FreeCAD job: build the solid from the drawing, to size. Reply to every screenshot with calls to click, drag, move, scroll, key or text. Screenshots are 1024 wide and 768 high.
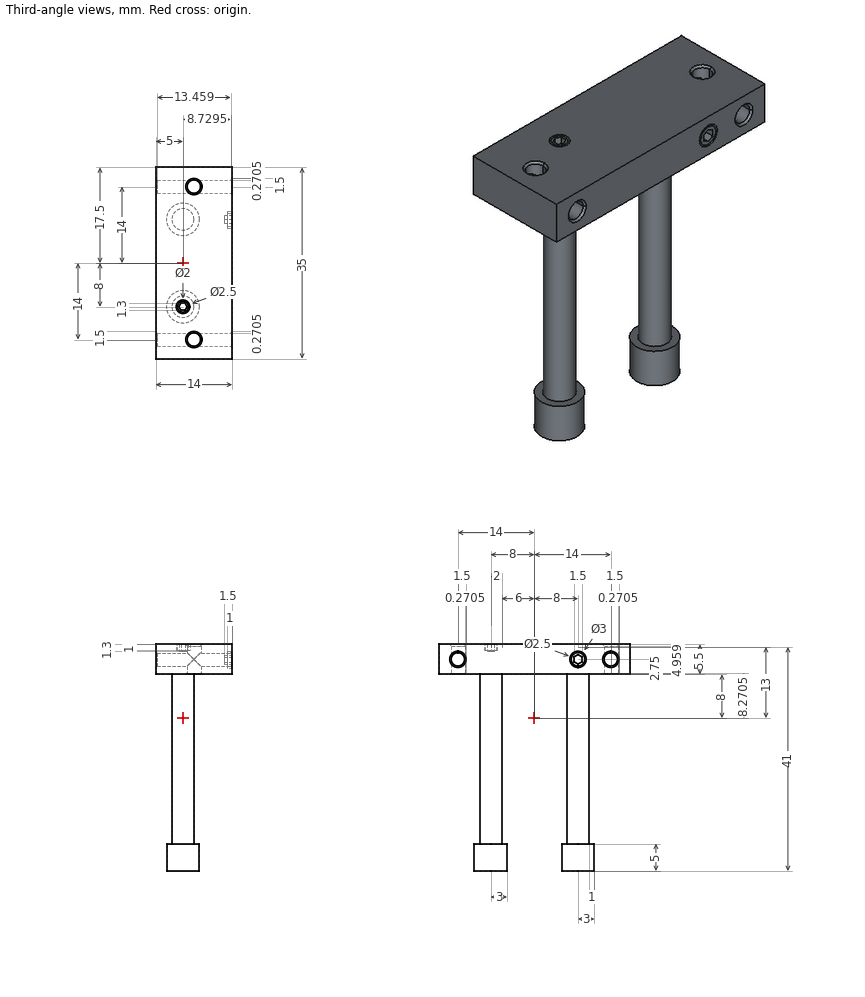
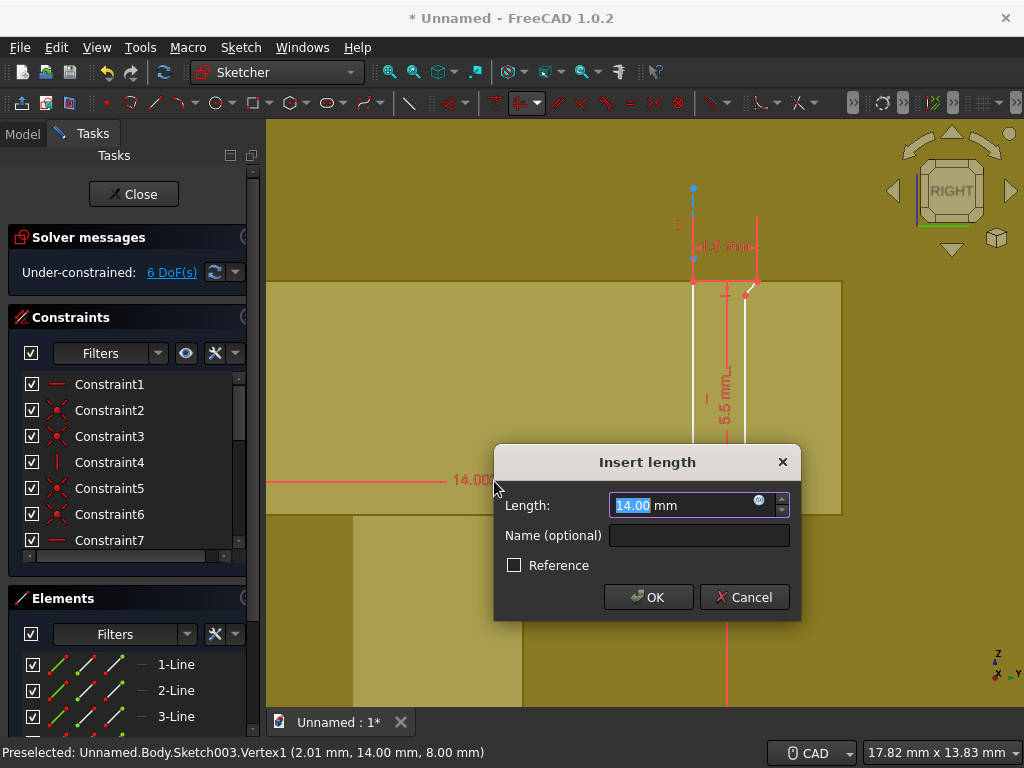
text(14)
key(Return)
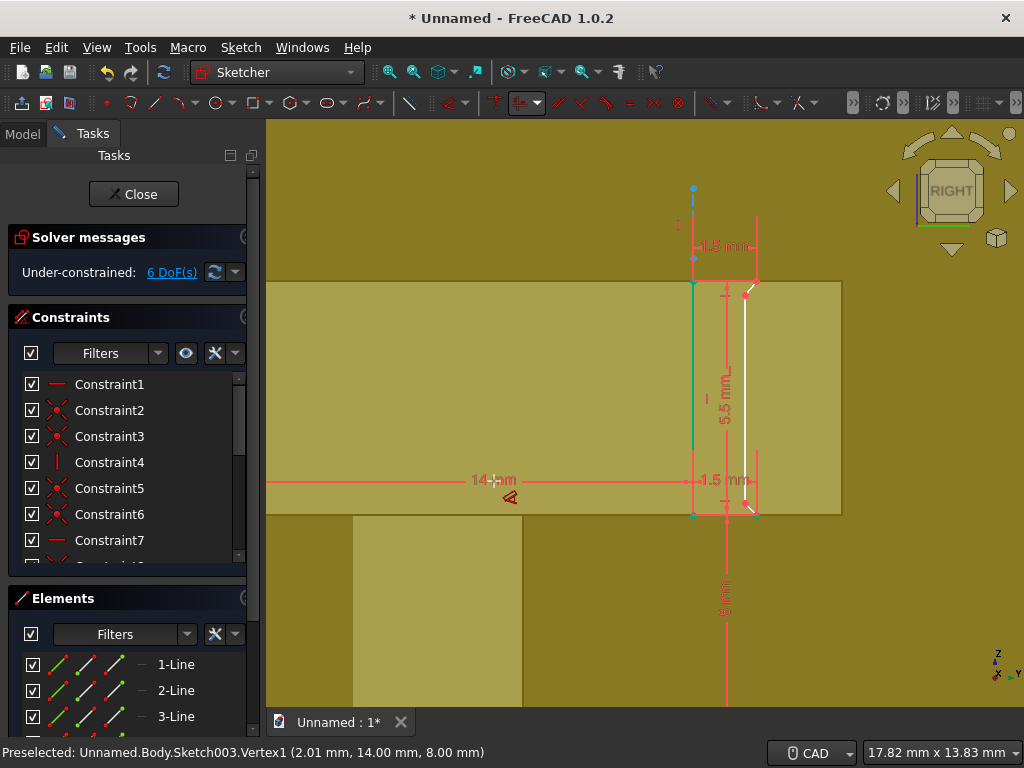
click(693, 259)
click(493, 225)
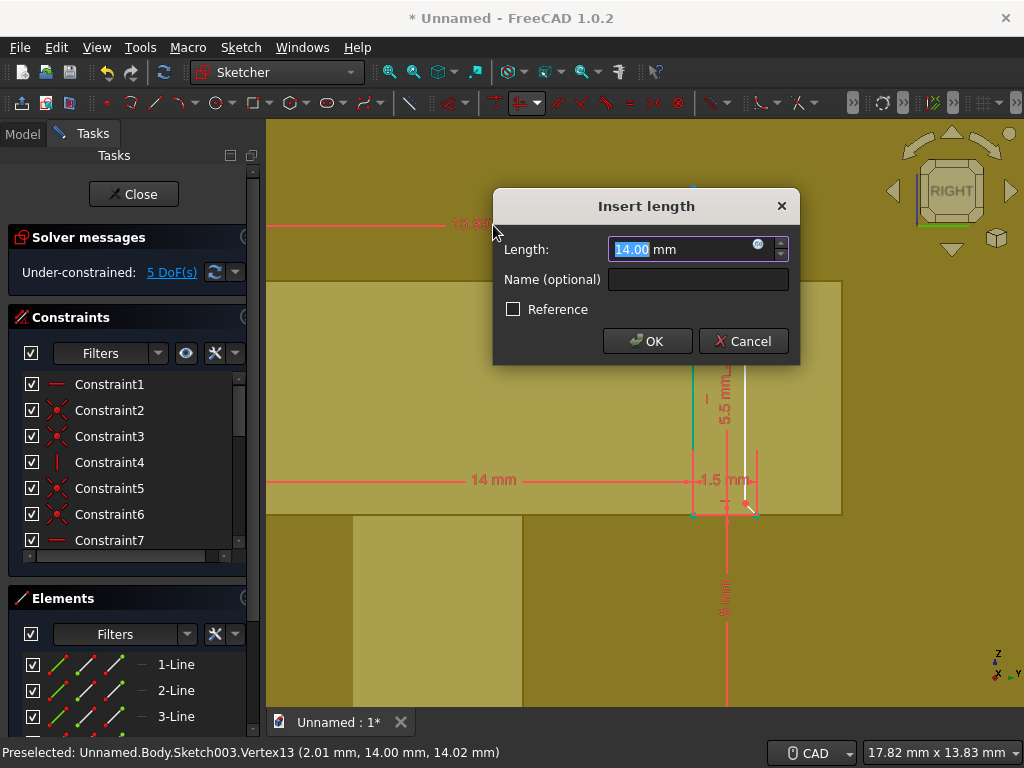
text(14)
key(Return)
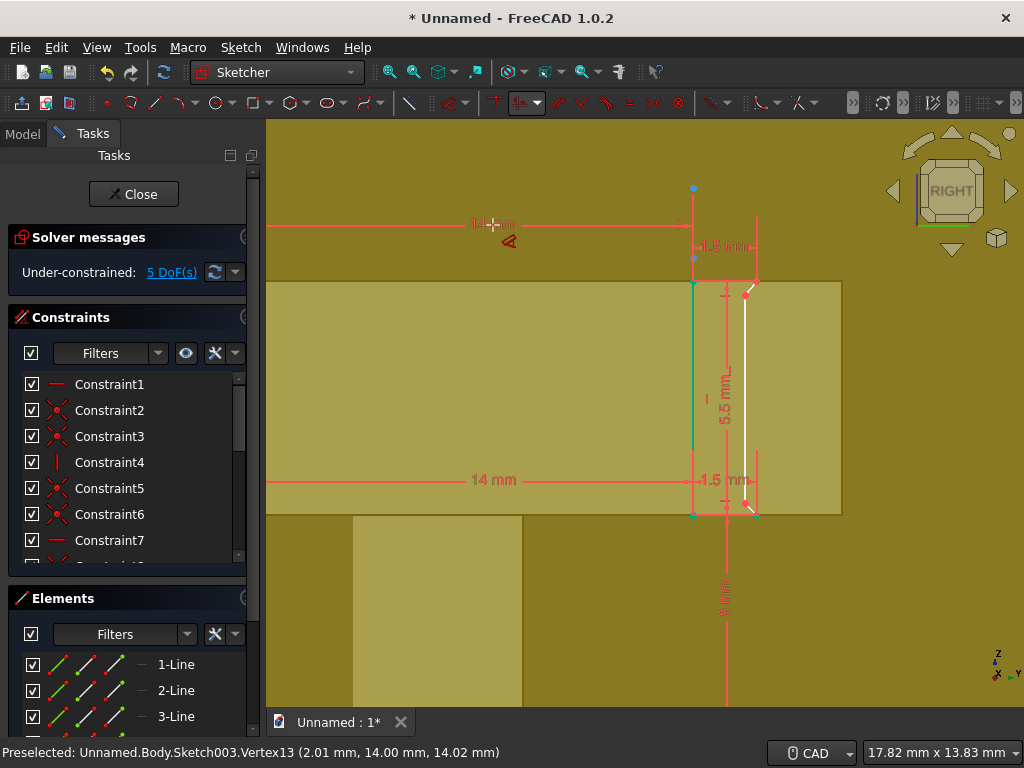
click(745, 441)
click(779, 352)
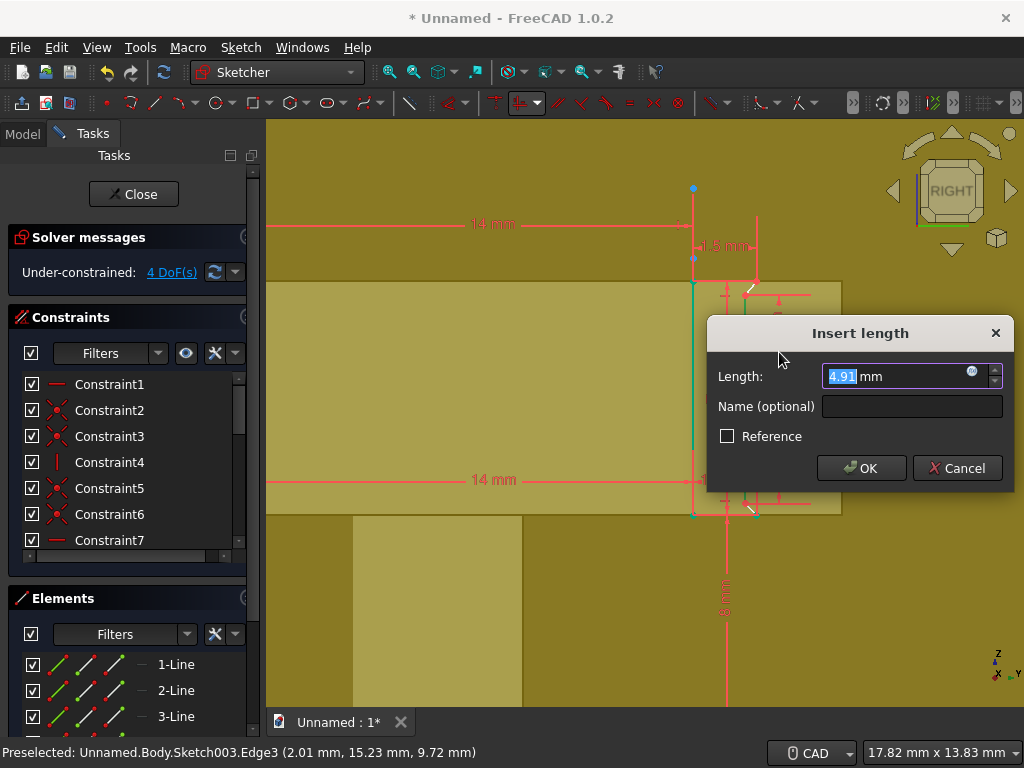
text(4.959)
key(Return)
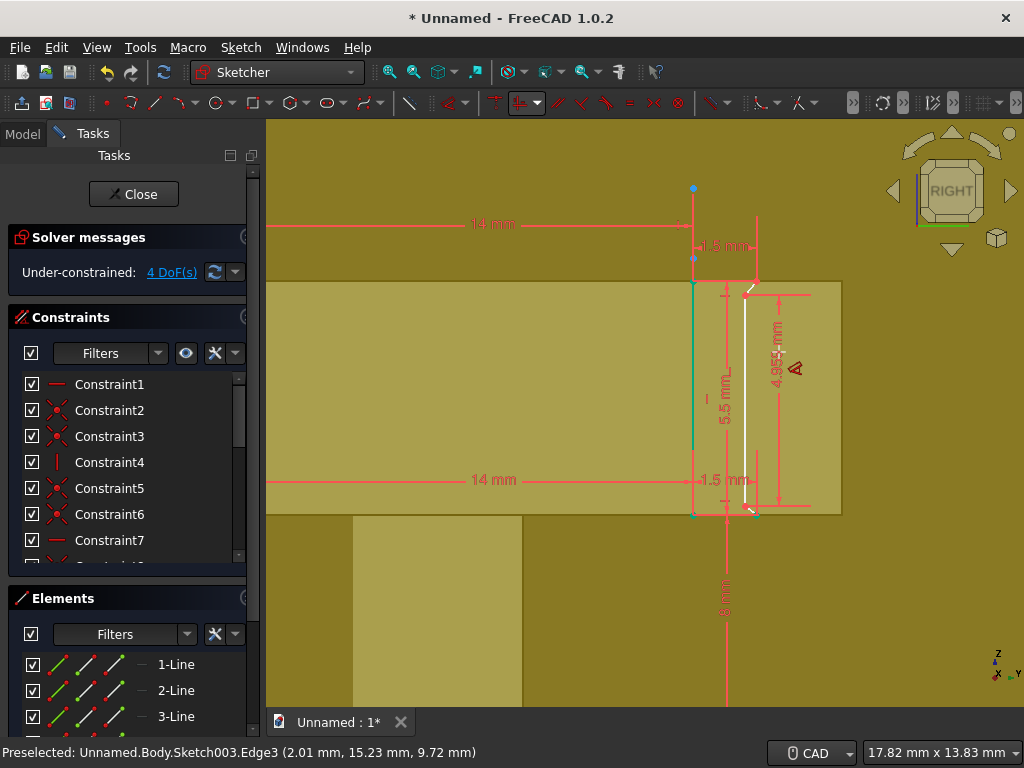
click(745, 506)
click(779, 553)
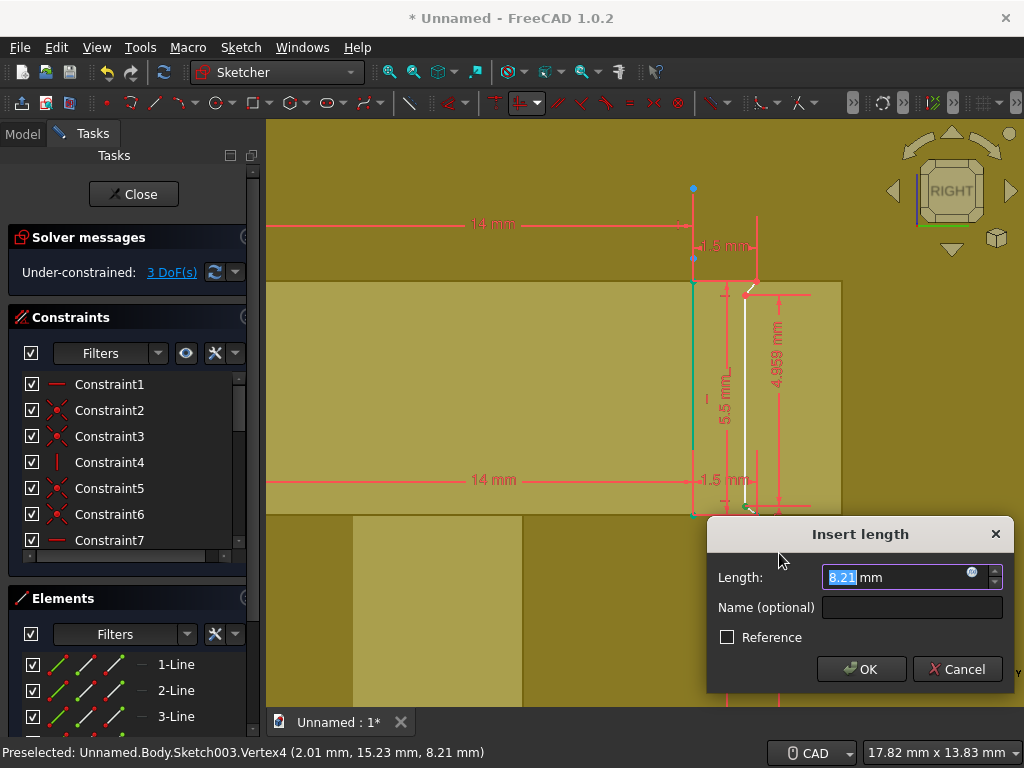
text(8.2705)
key(Return)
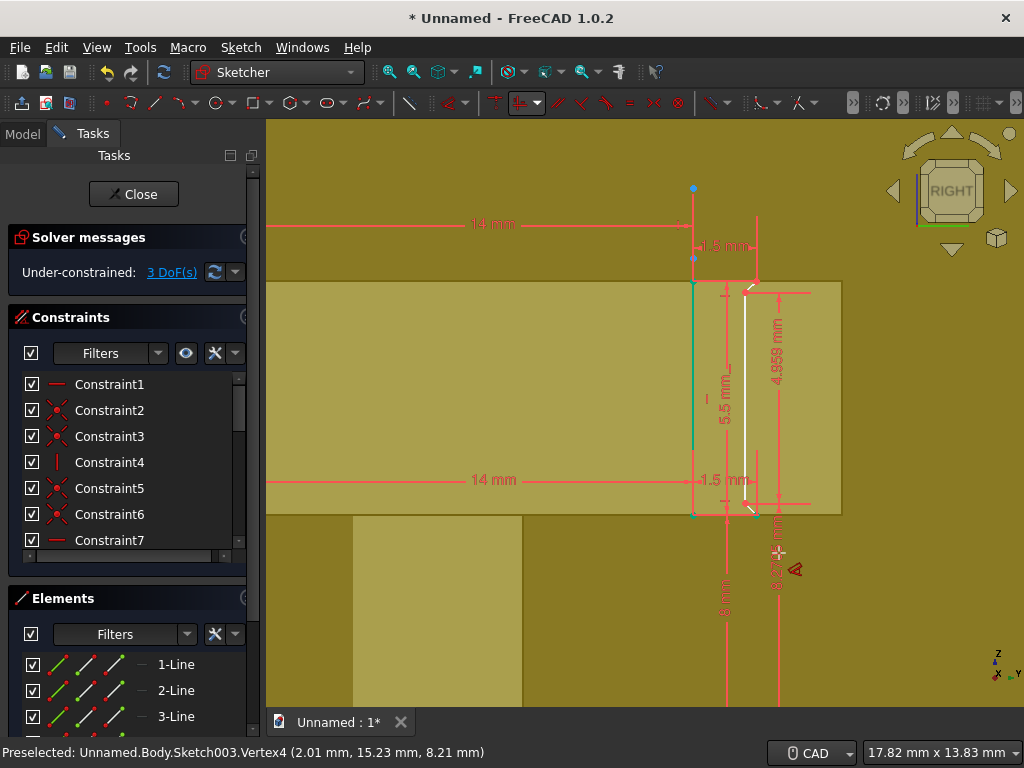
scroll(750, 508, up, 7)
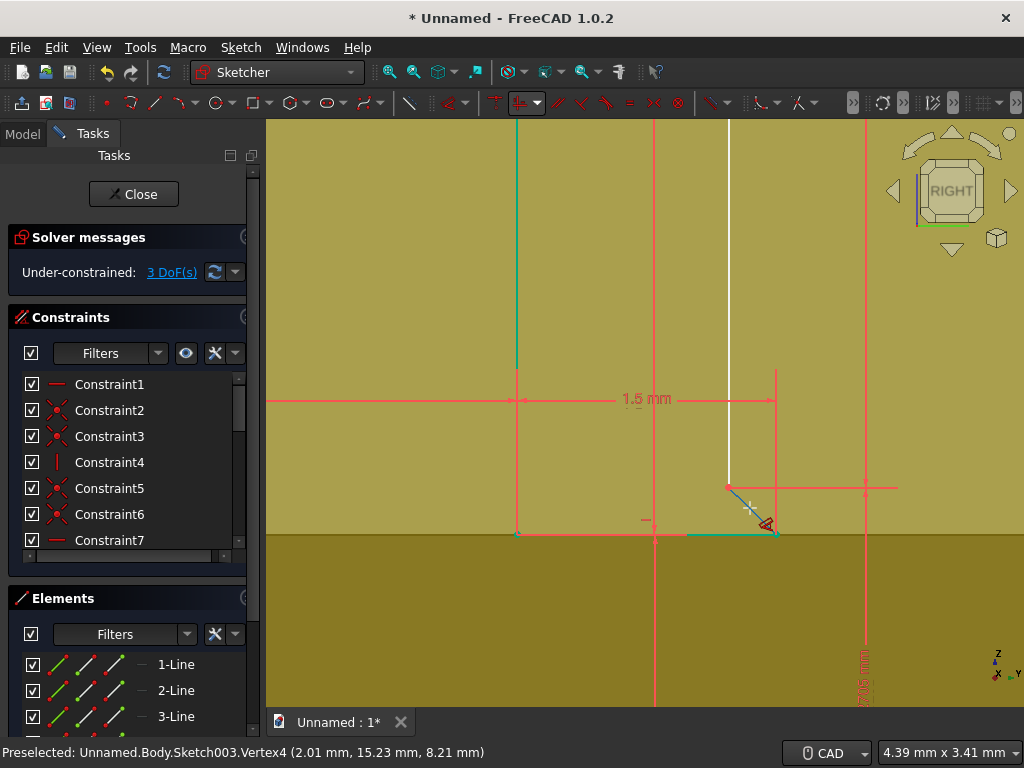
click(748, 507)
click(752, 454)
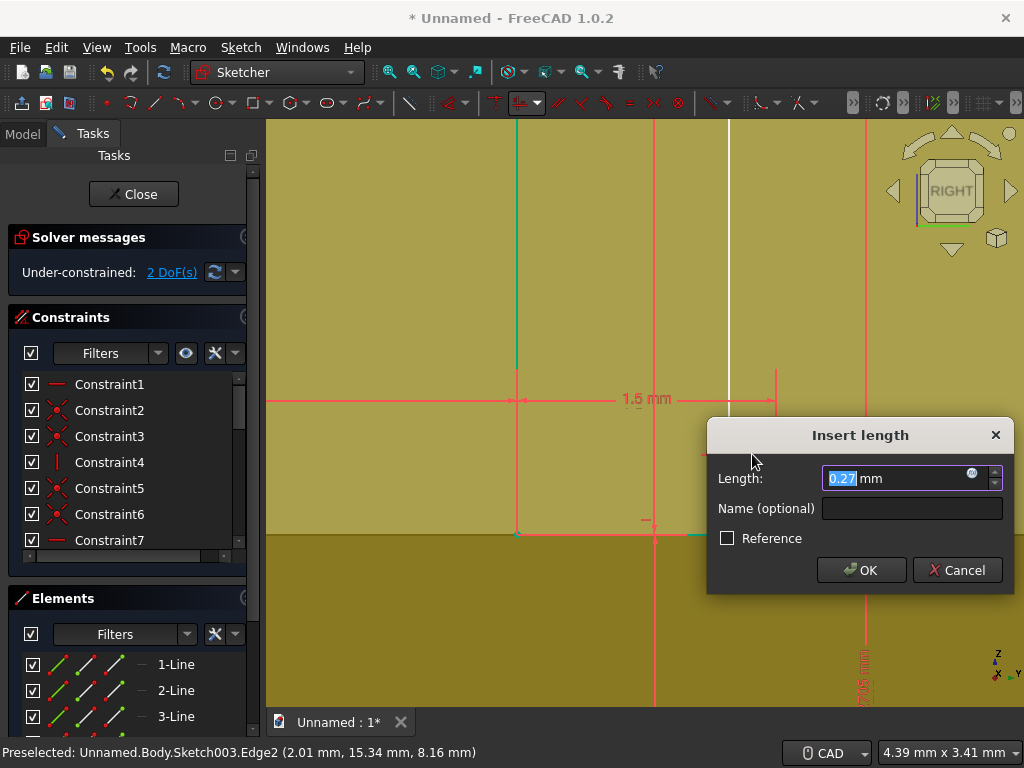
text(0.2705)
key(Return)
key(Escape)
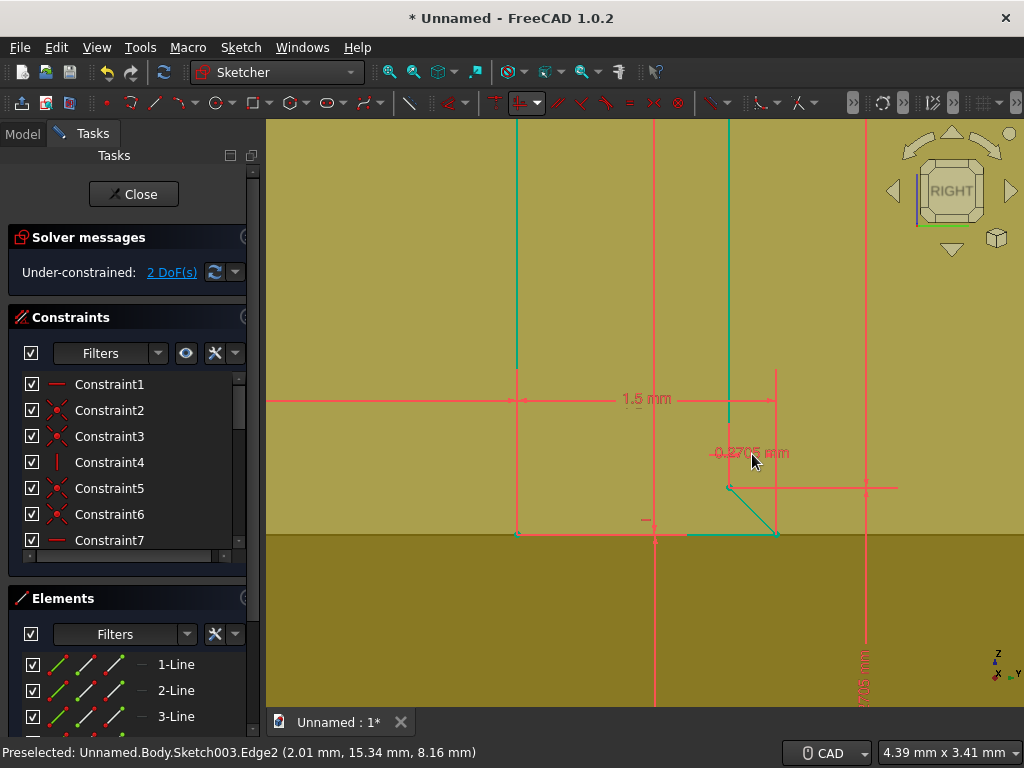
click(134, 194)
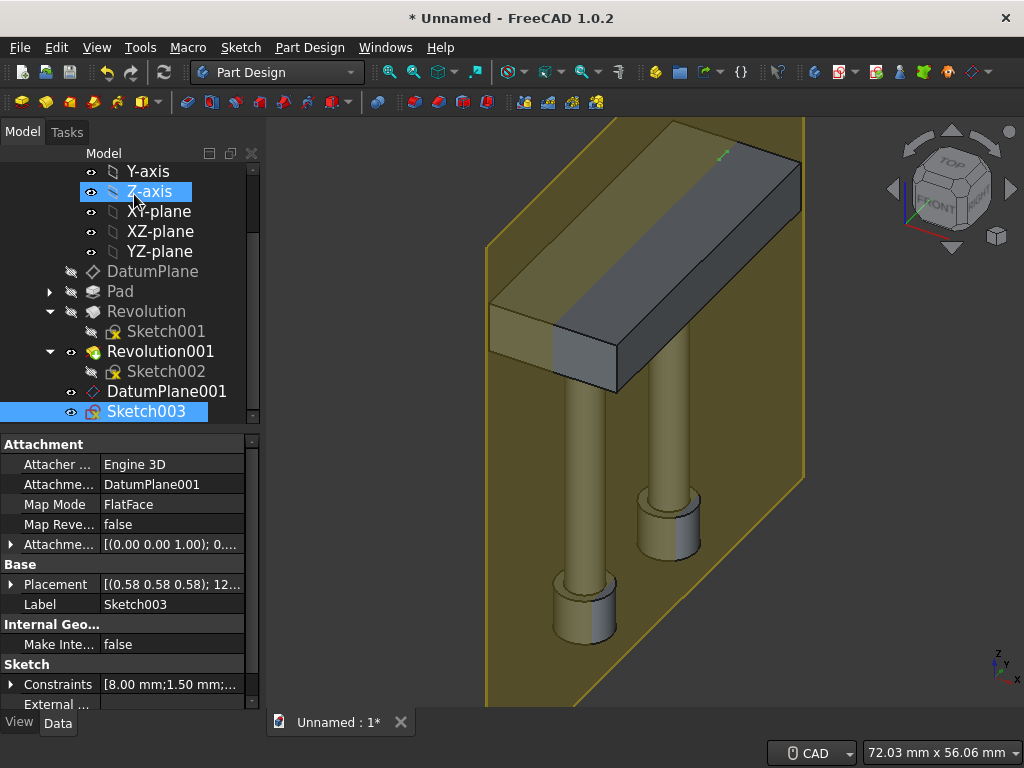
click(236, 102)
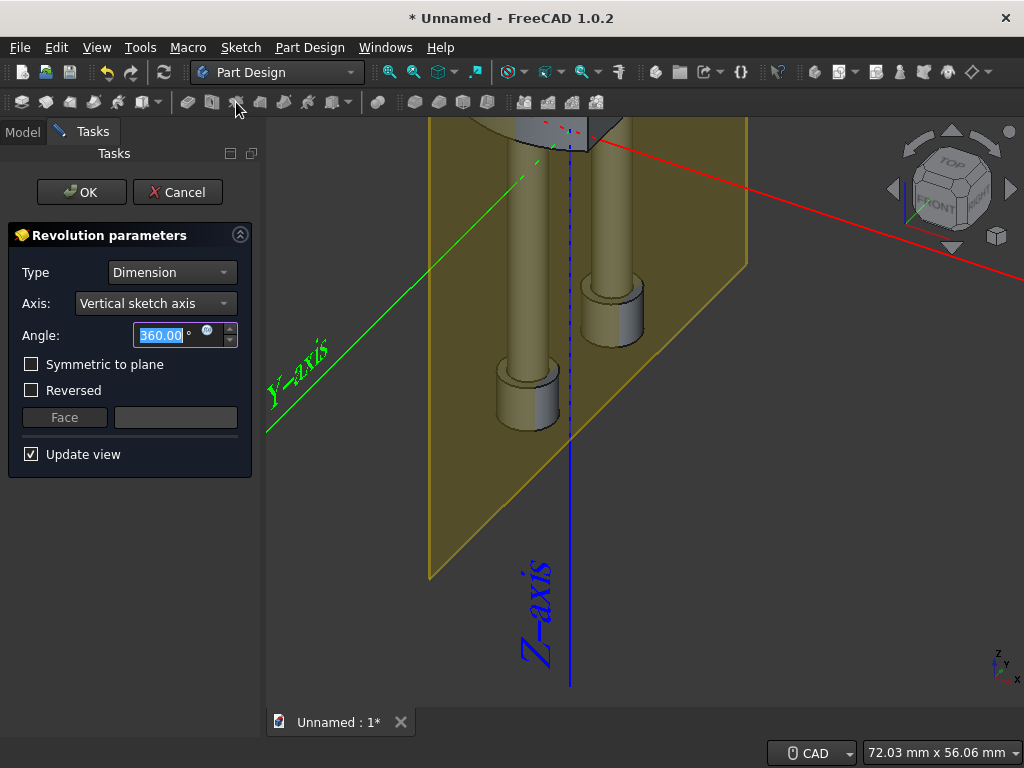
click(156, 304)